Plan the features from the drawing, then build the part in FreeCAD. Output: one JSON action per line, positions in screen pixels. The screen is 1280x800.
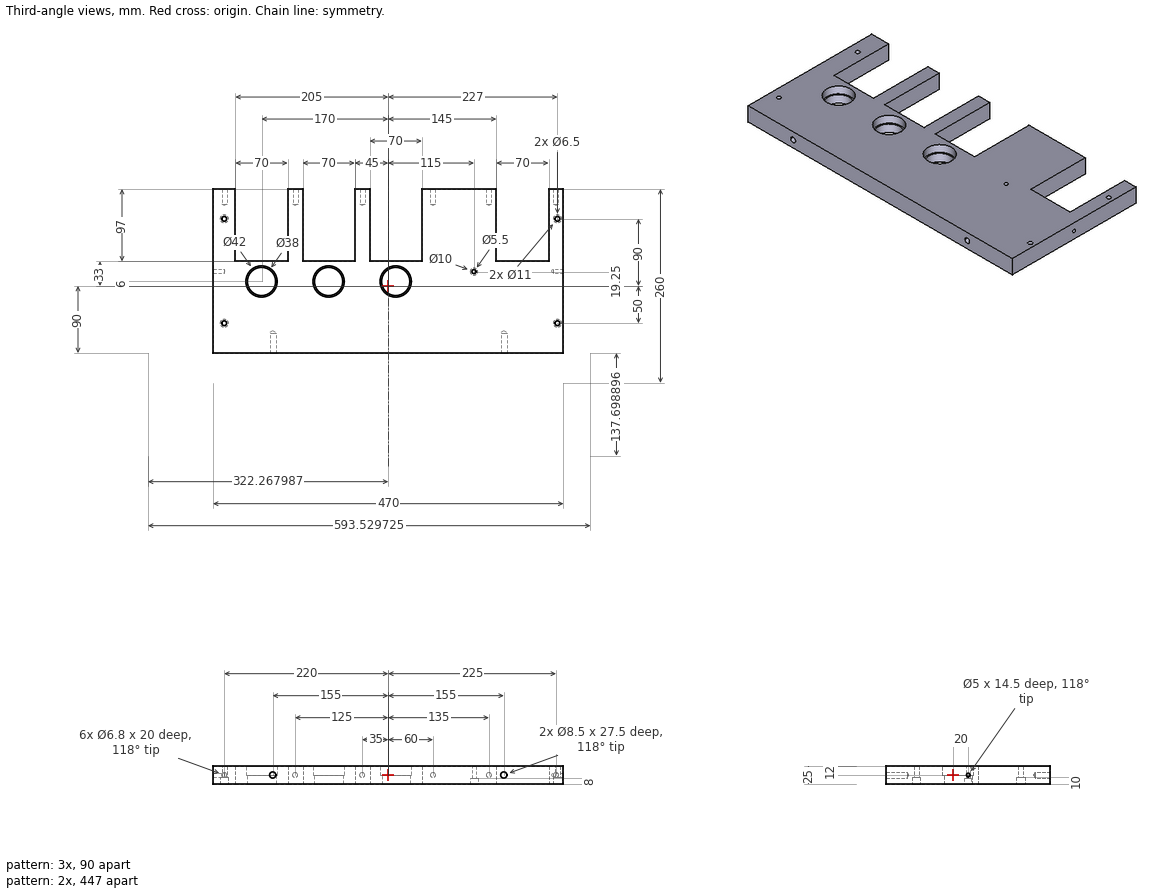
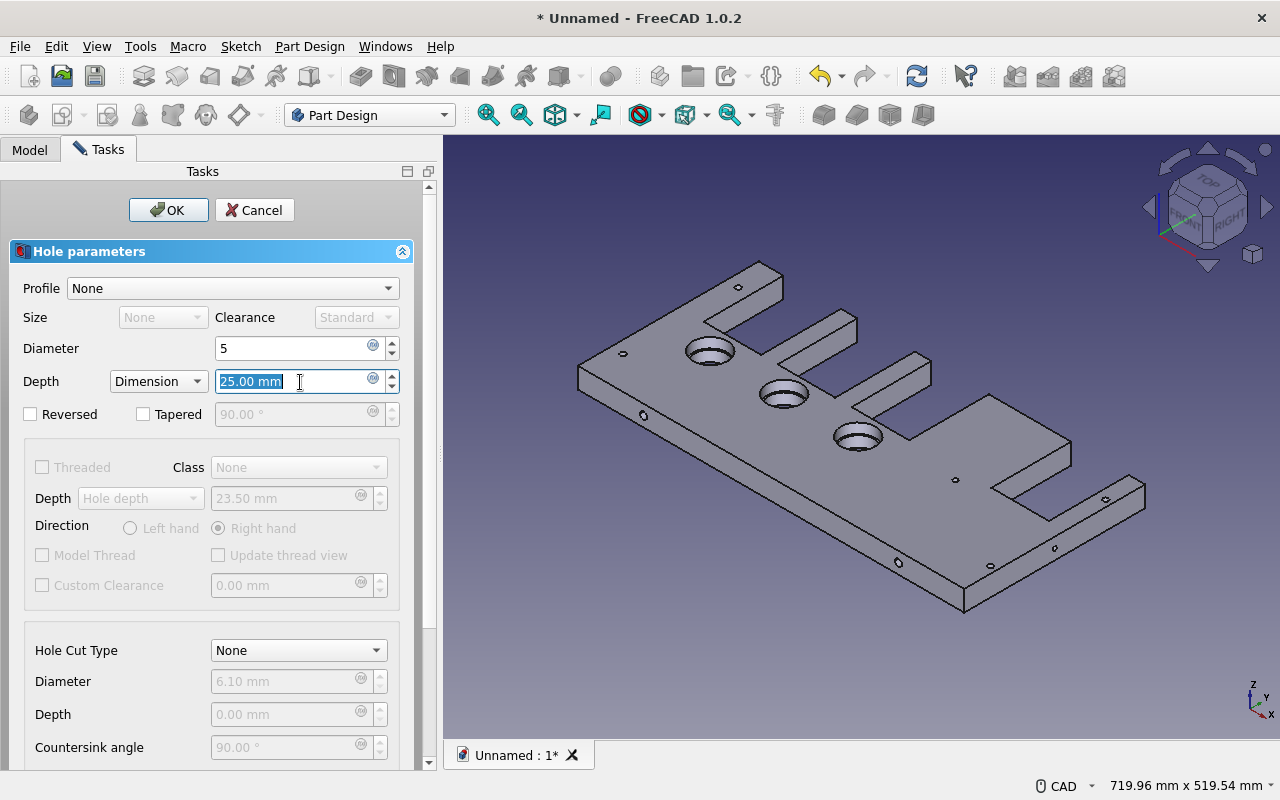
{"action": "type", "text": "14.5"}
{"action": "key", "text": "Tab"}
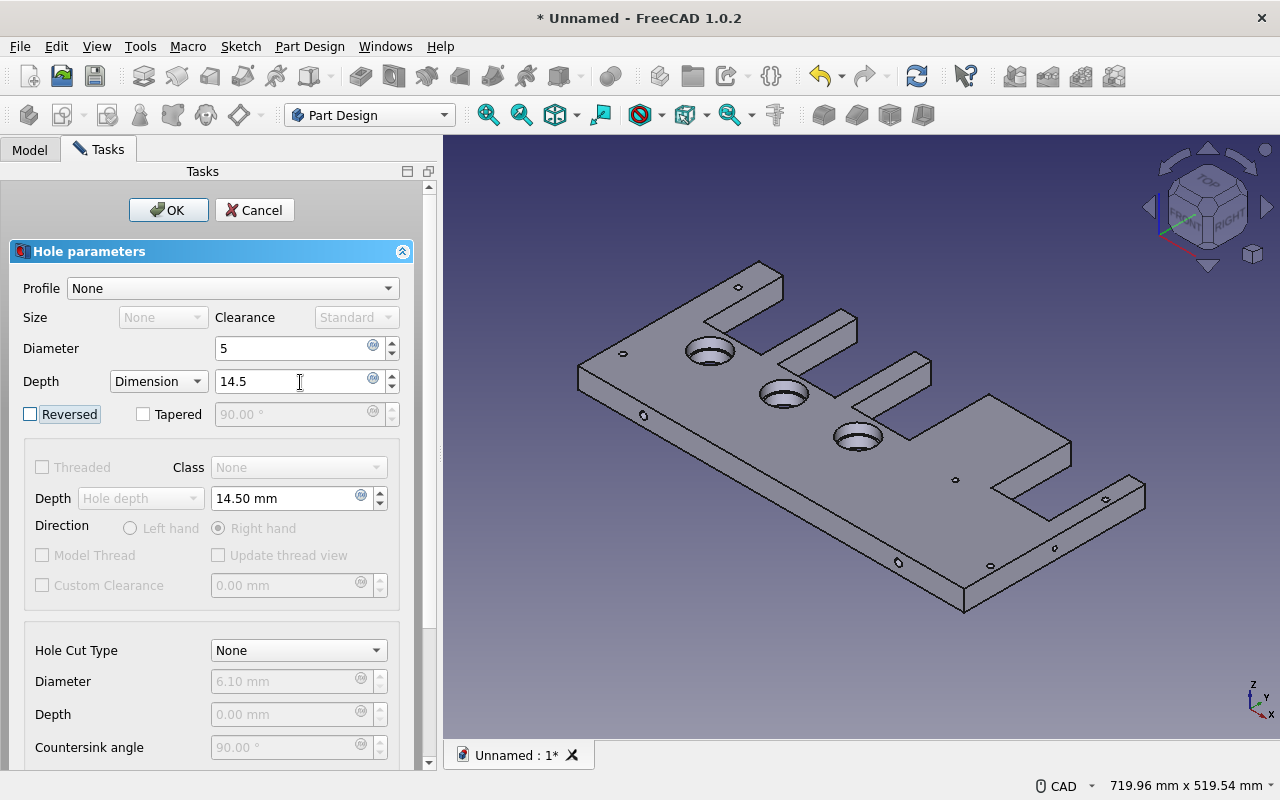
{"action": "left_click", "coordinate": [169, 210]}